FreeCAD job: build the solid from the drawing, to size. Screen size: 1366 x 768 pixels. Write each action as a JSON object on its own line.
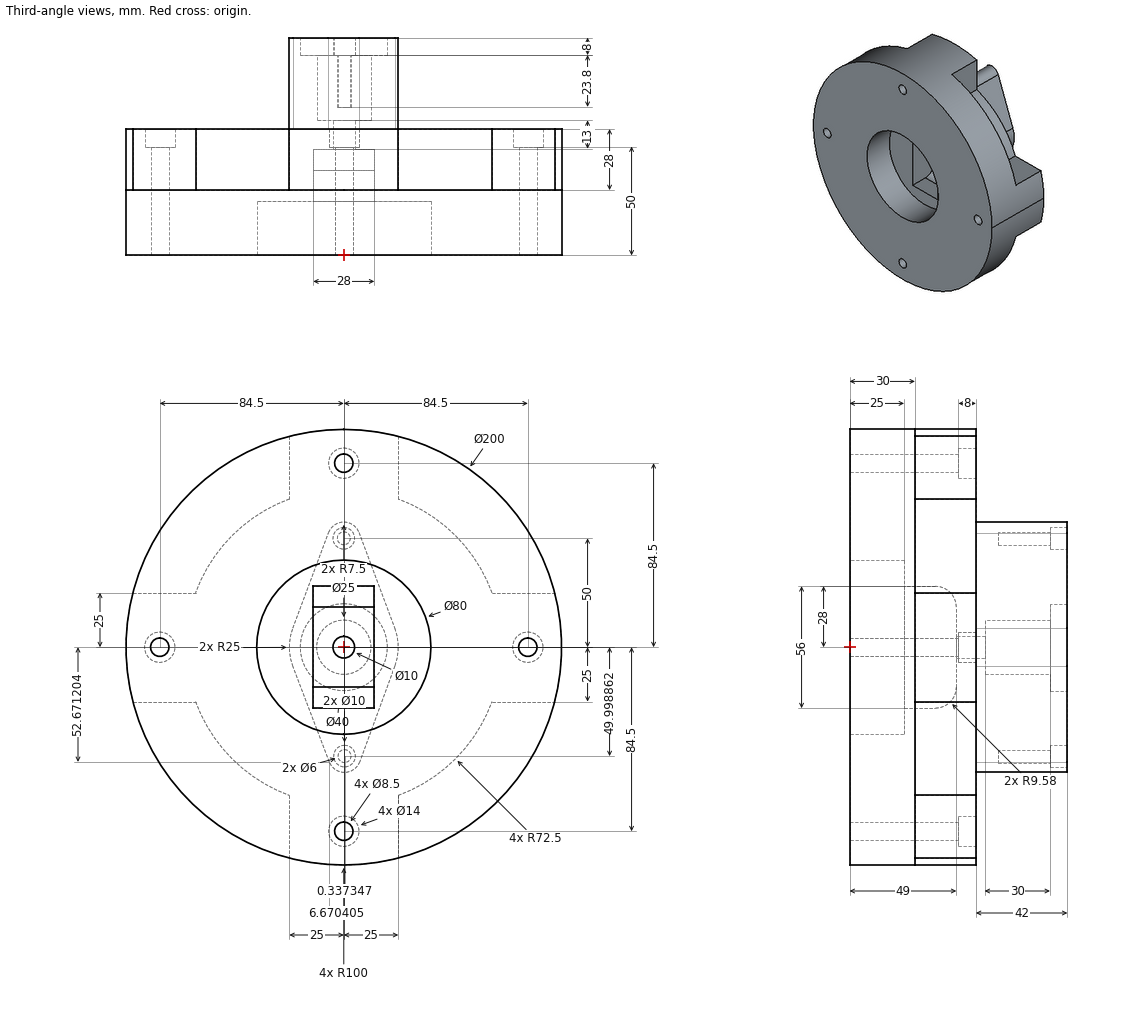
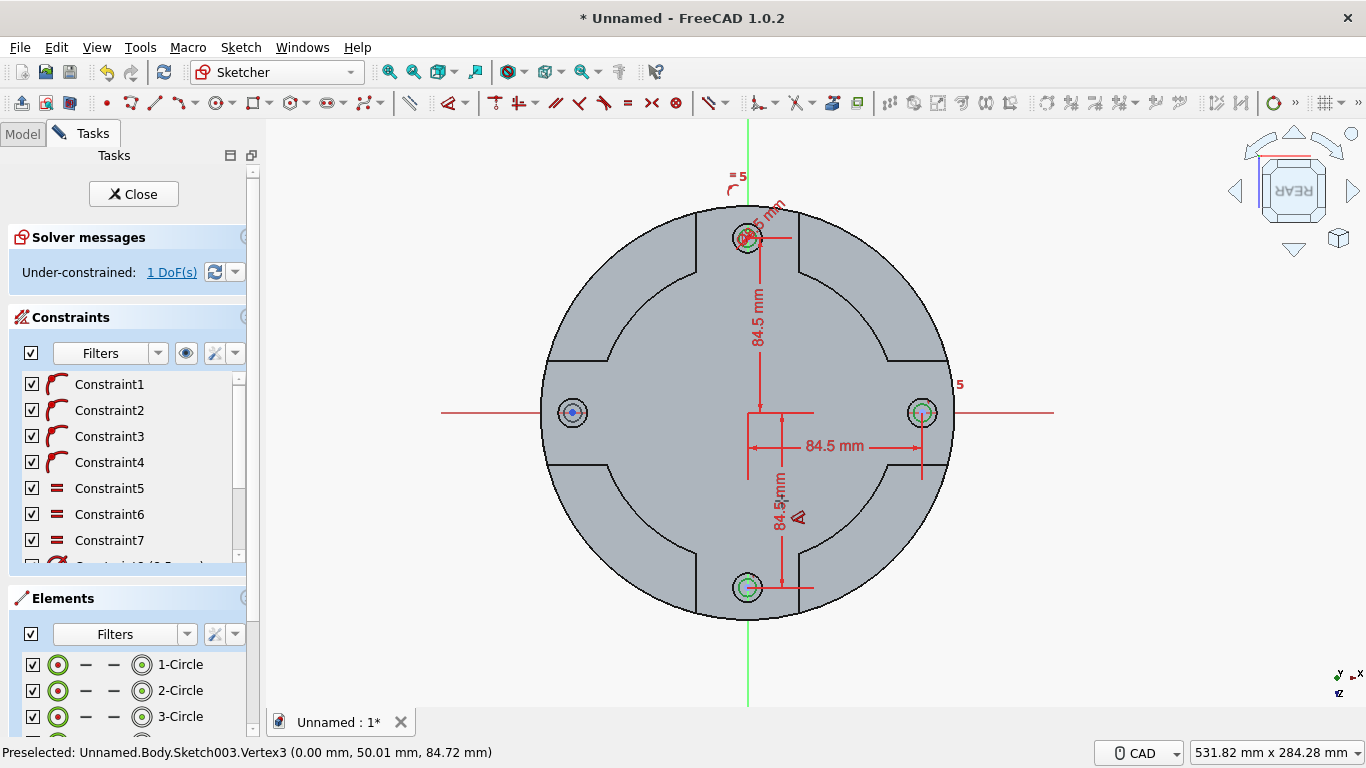
{"action": "left_click", "coordinate": [573, 413]}
{"action": "left_click", "coordinate": [660, 447]}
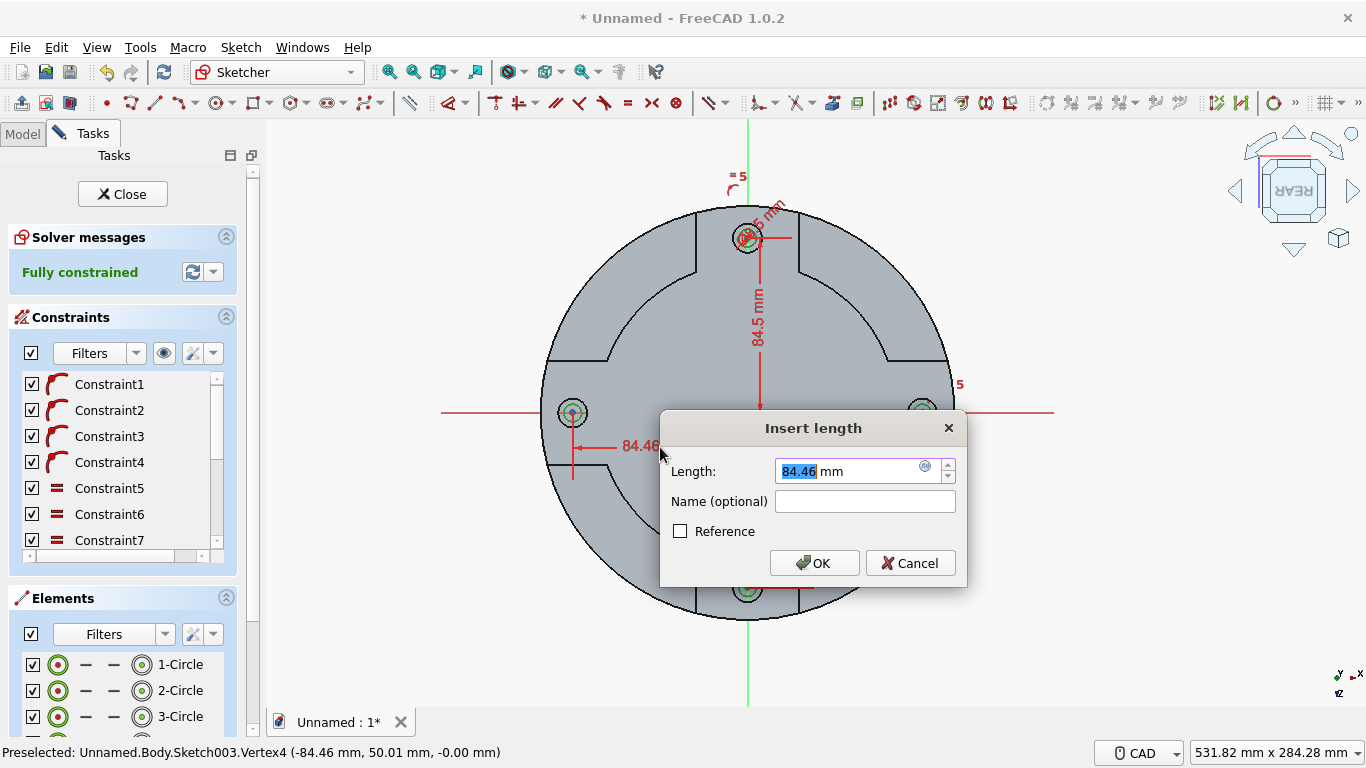
{"action": "type", "text": "84.5"}
{"action": "key", "text": "Return"}
{"action": "key", "text": "Escape"}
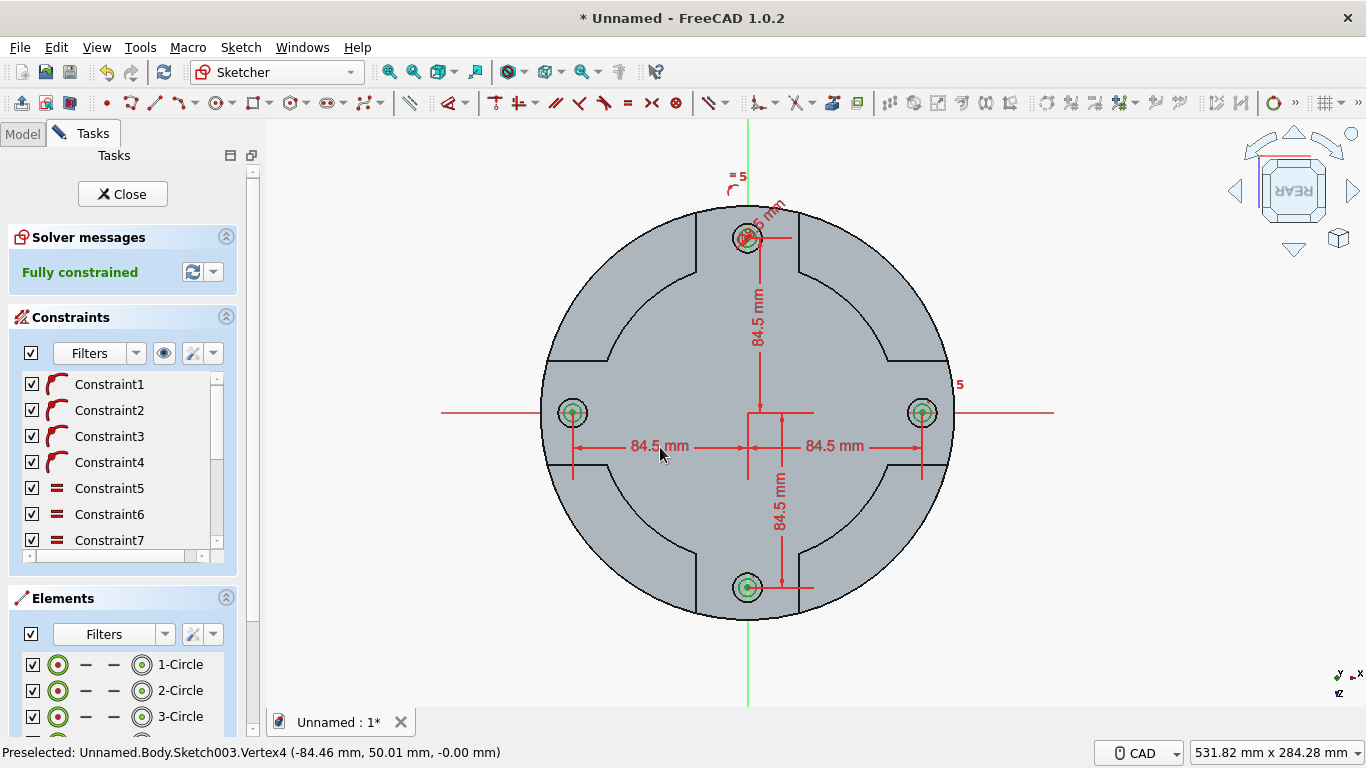
{"action": "left_click", "coordinate": [123, 194]}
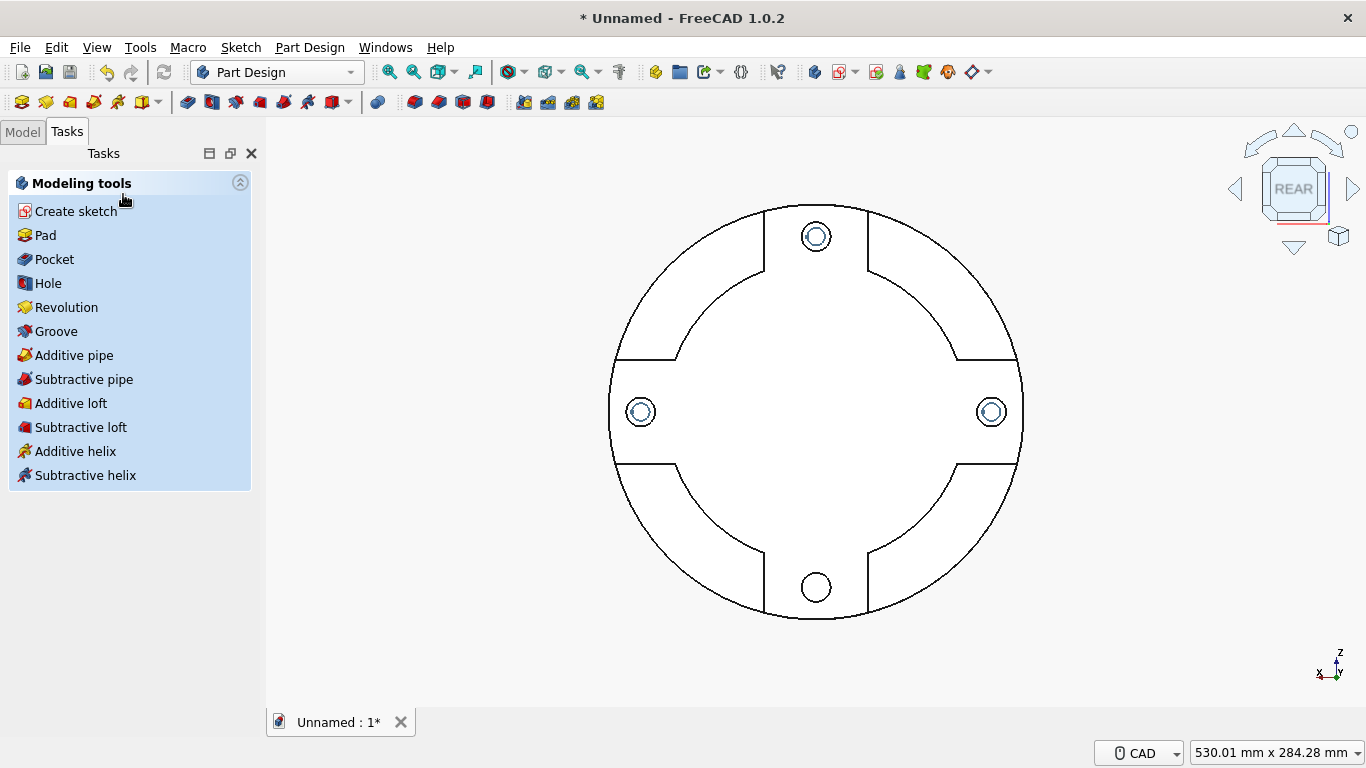
{"action": "left_click", "coordinate": [188, 102]}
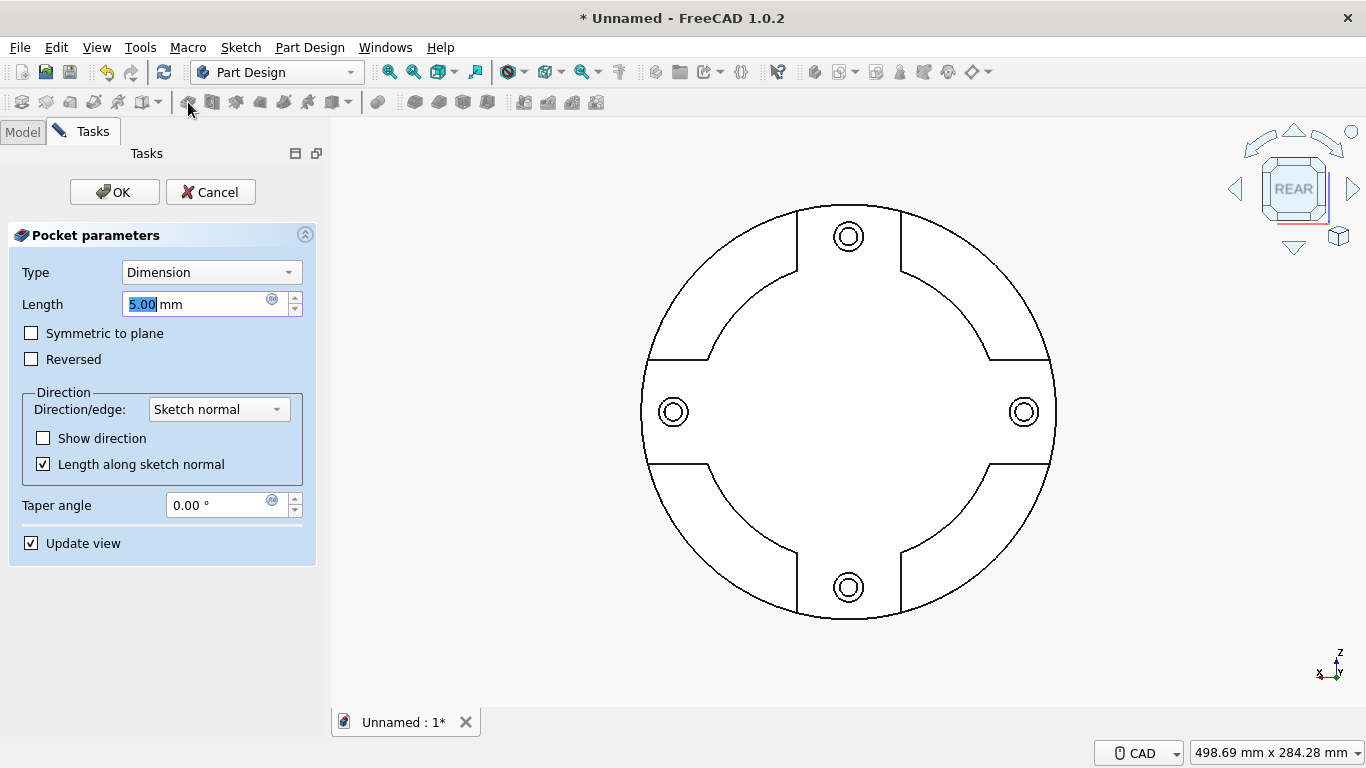
{"action": "type", "text": "50"}
{"action": "key", "text": "Tab"}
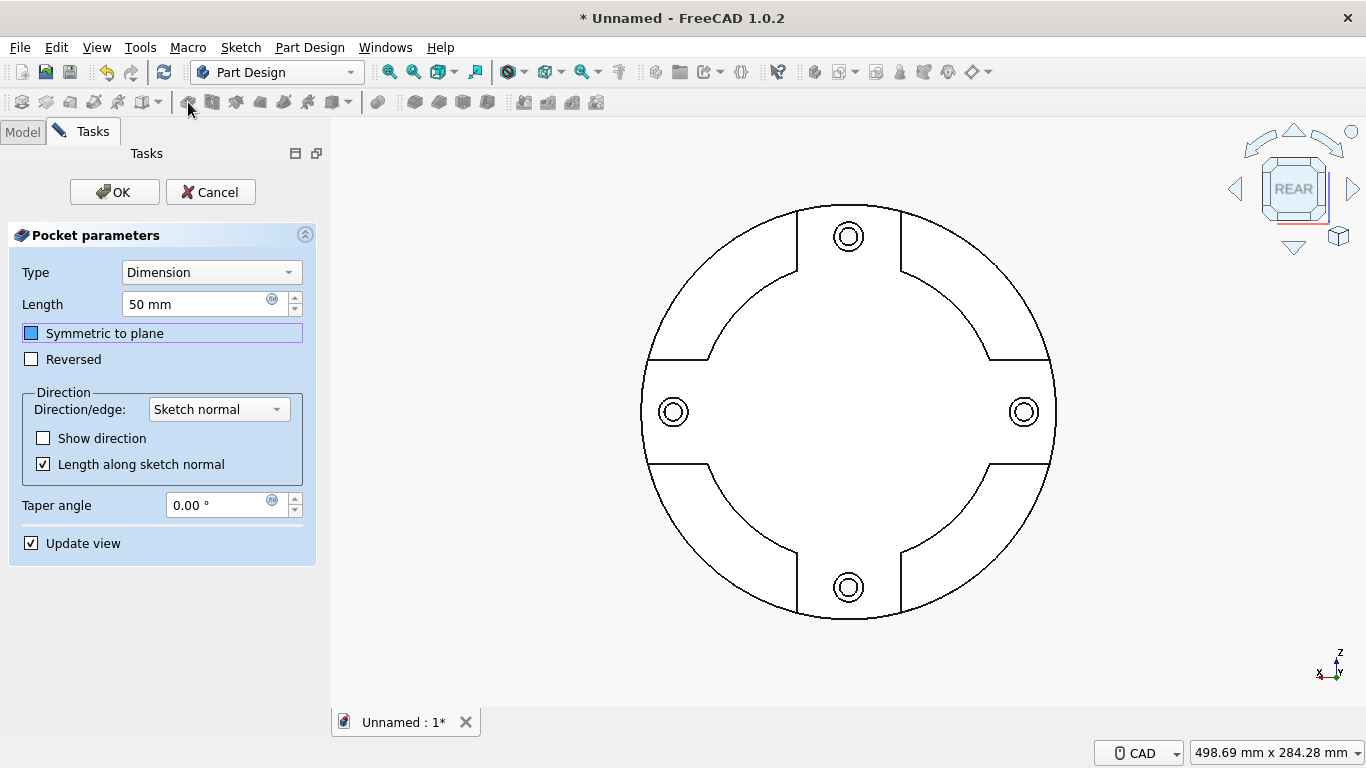
{"action": "left_click", "coordinate": [115, 192]}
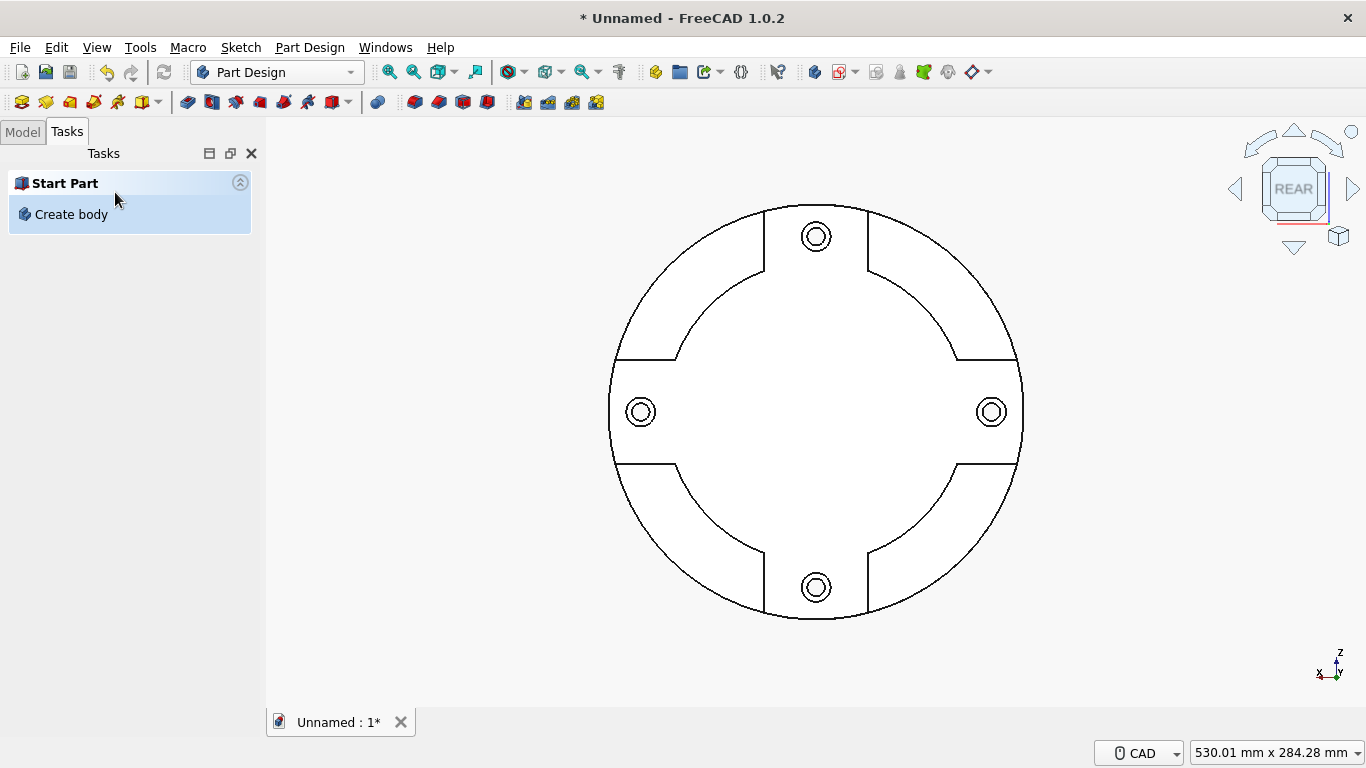
{"action": "left_click", "coordinate": [816, 411]}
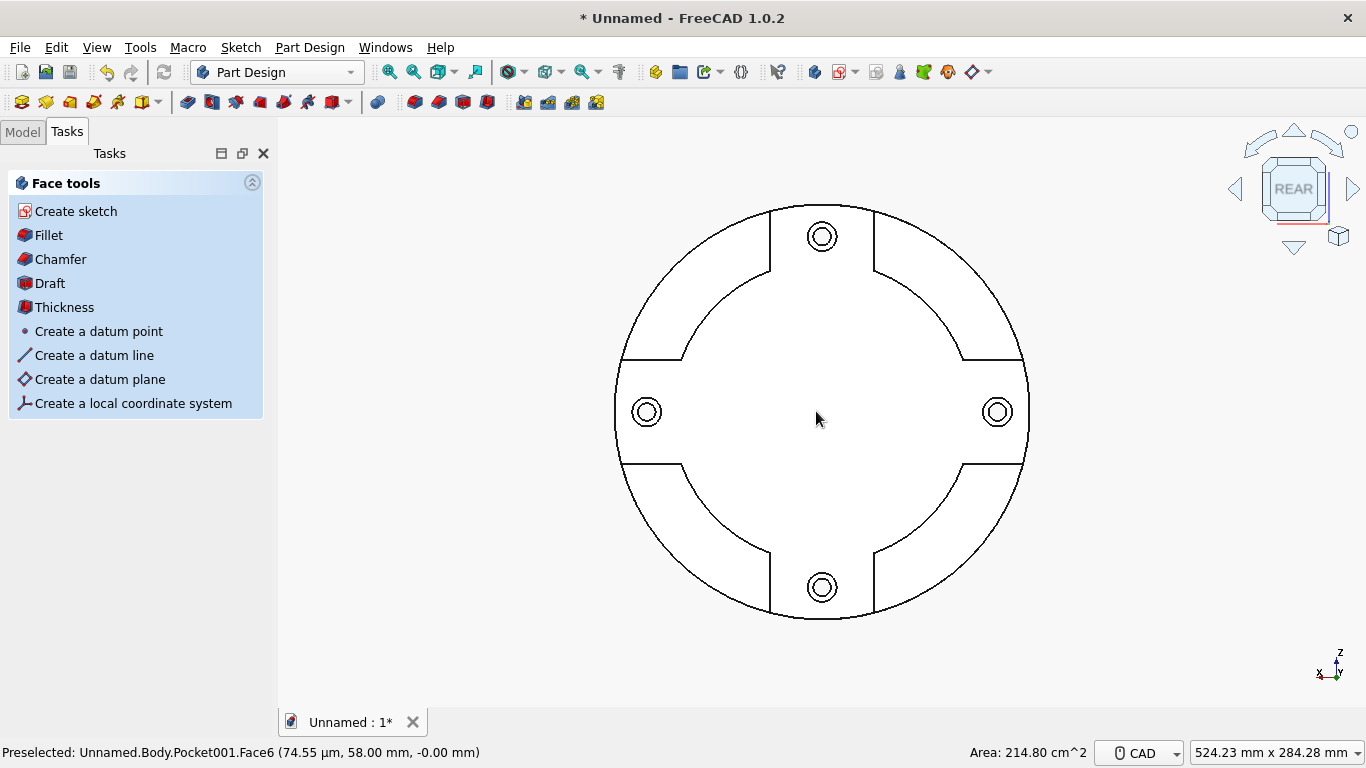
{"action": "left_click", "coordinate": [840, 72]}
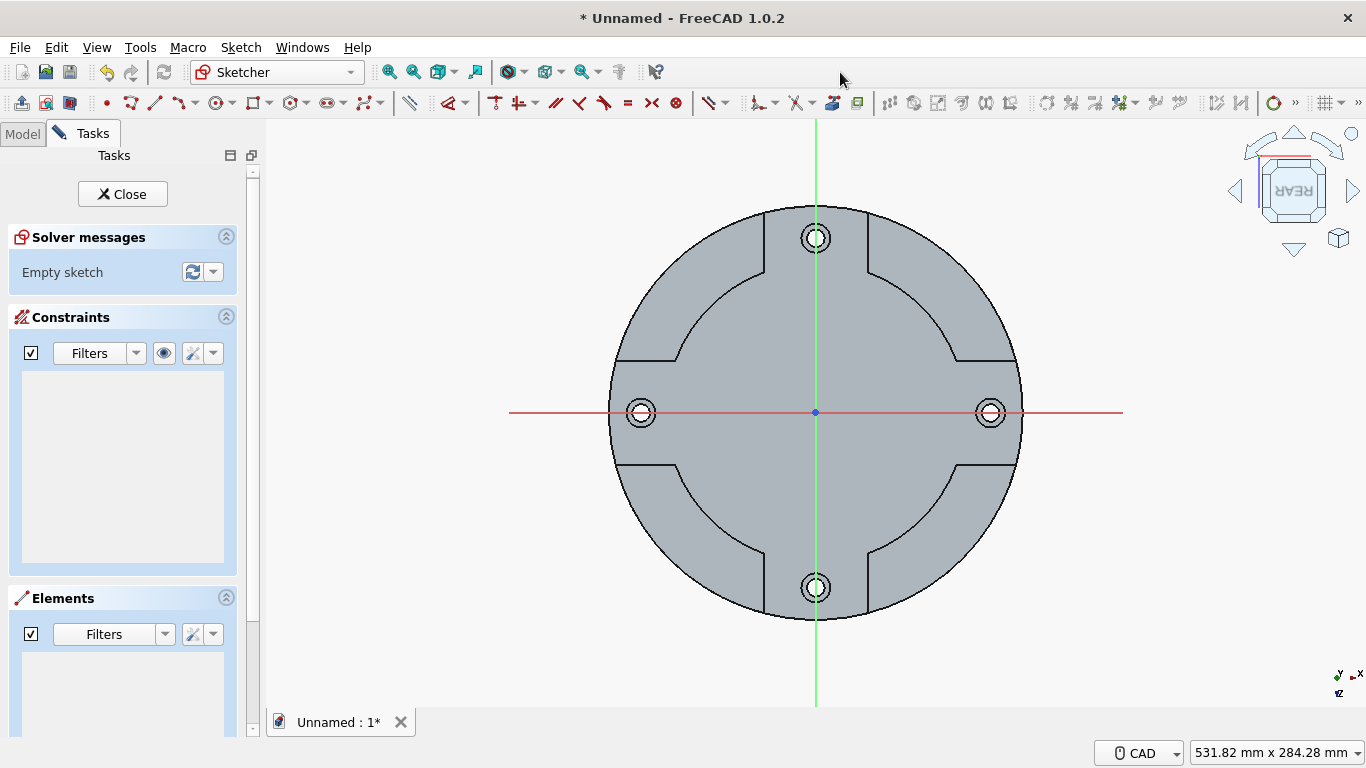
{"action": "scroll", "coordinate": [955, 413], "scroll_direction": "up", "scroll_amount": 2}